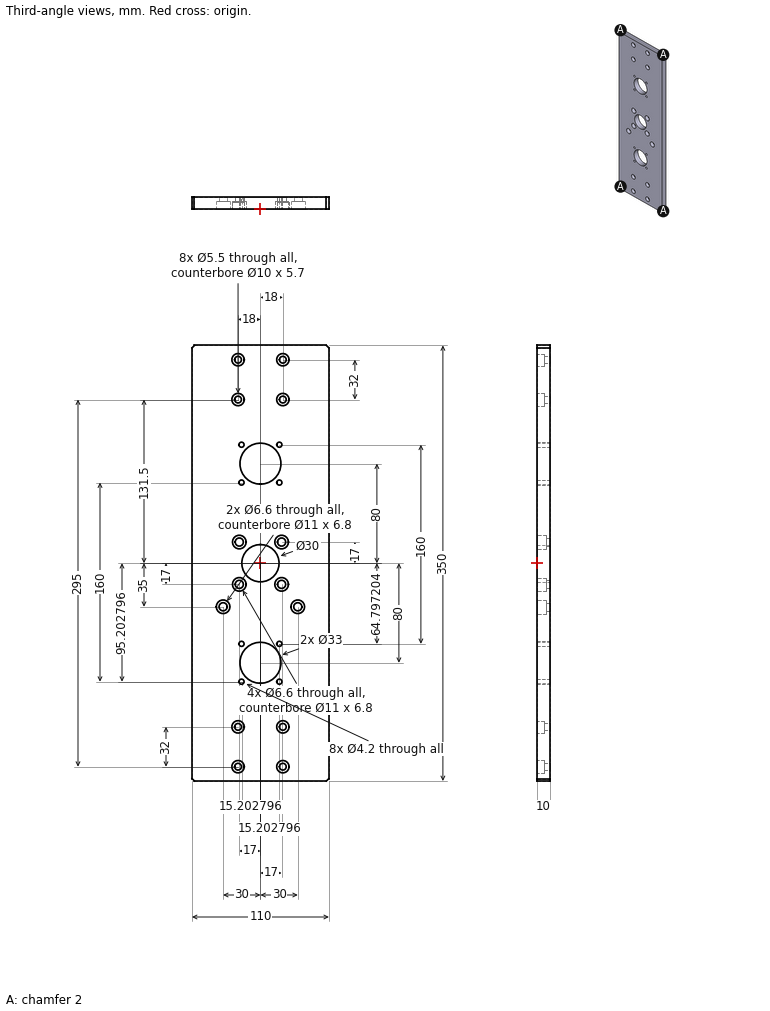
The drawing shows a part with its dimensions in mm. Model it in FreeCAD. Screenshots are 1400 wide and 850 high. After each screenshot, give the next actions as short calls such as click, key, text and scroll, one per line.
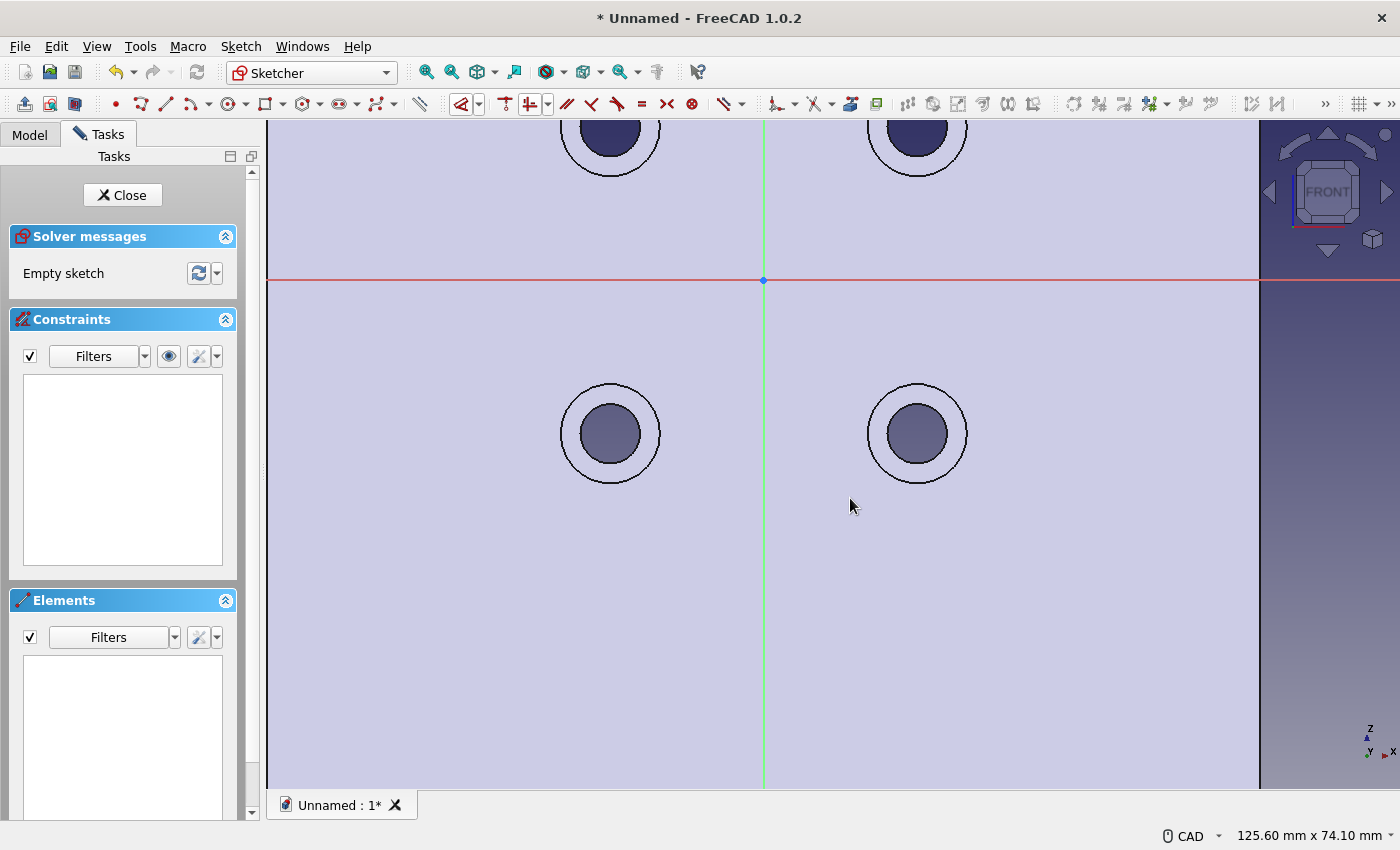
key(g)
key(c)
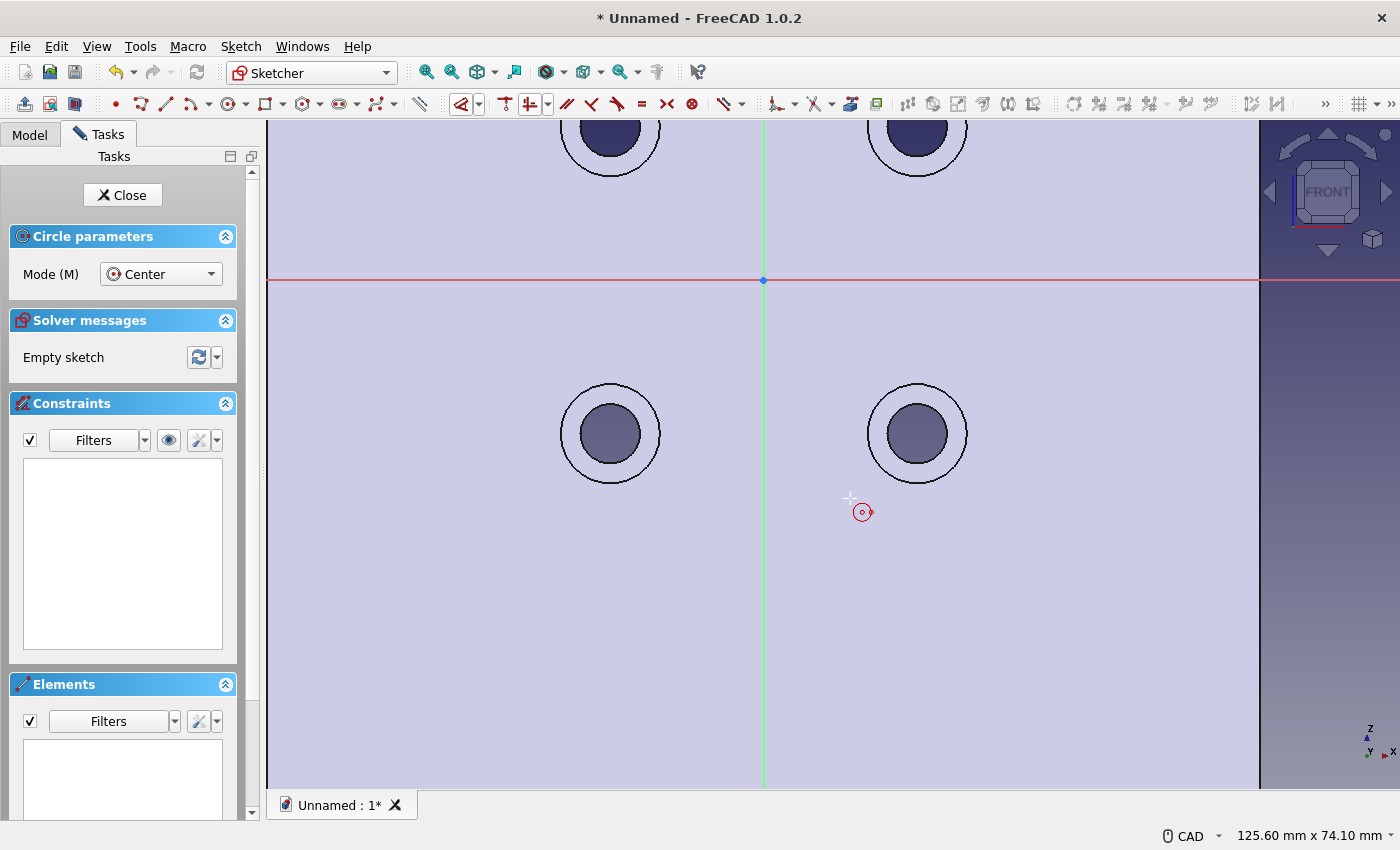
click(493, 596)
move(514, 575)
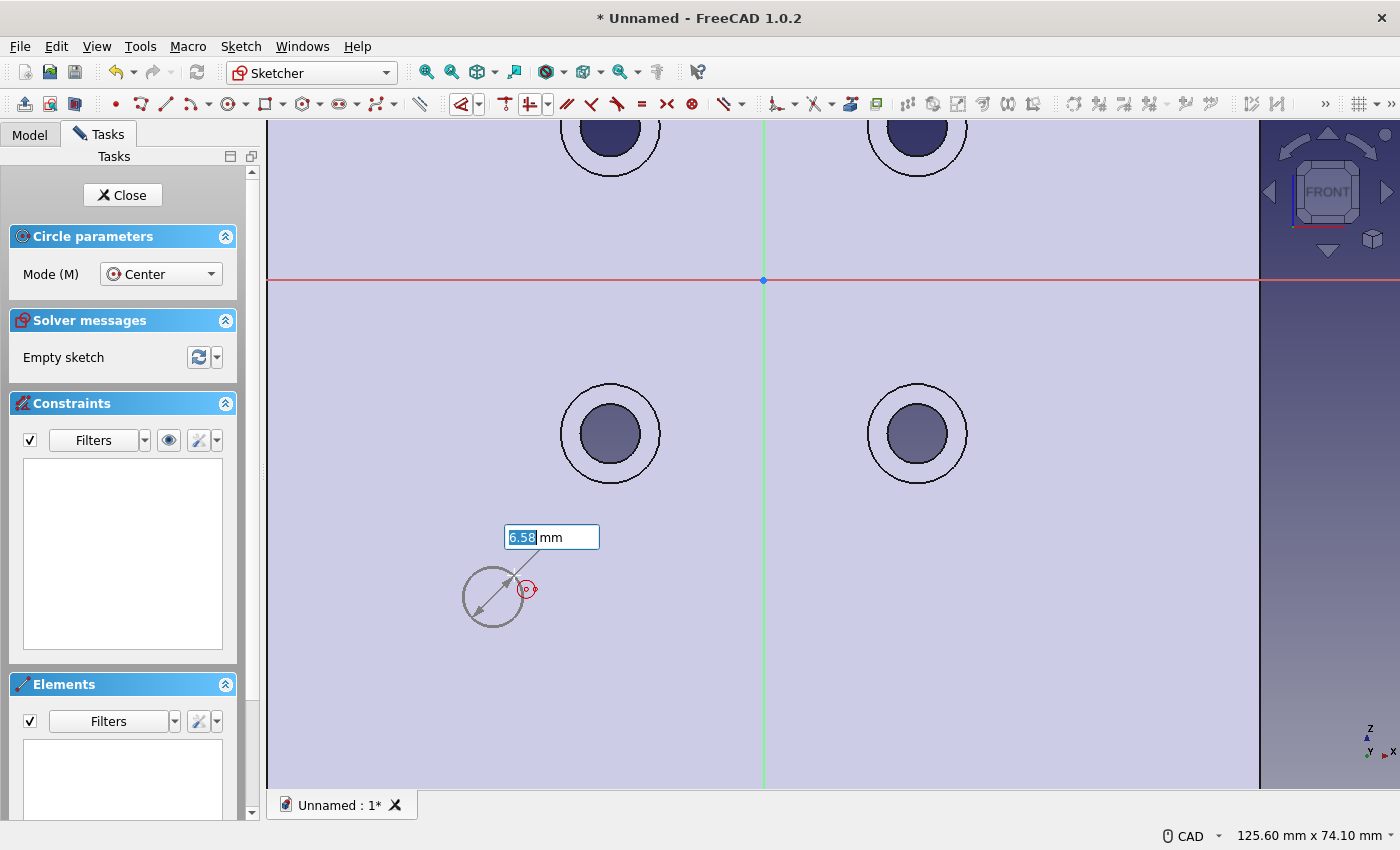
text(6.6)
key(Return)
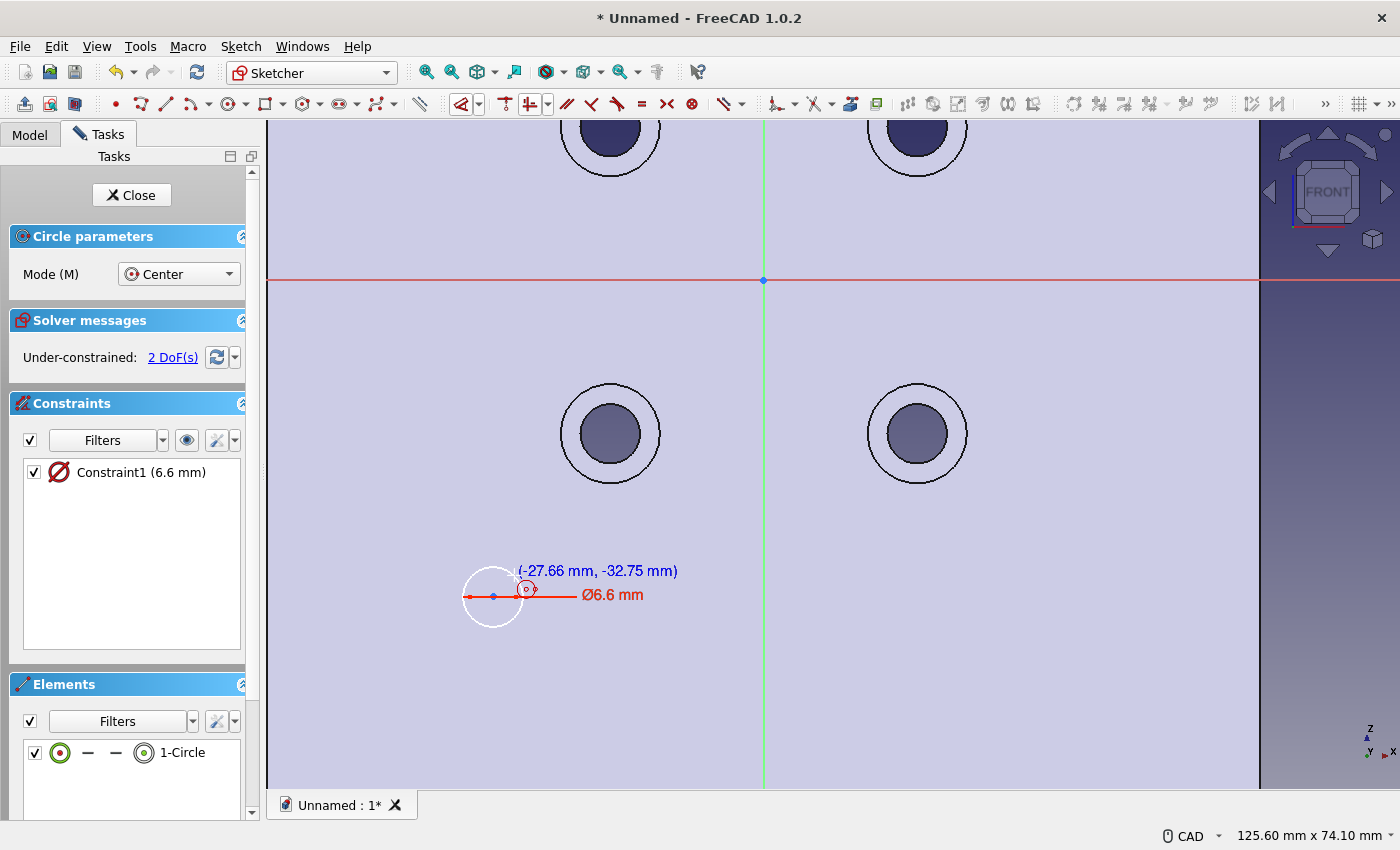
click(1035, 596)
move(1056, 575)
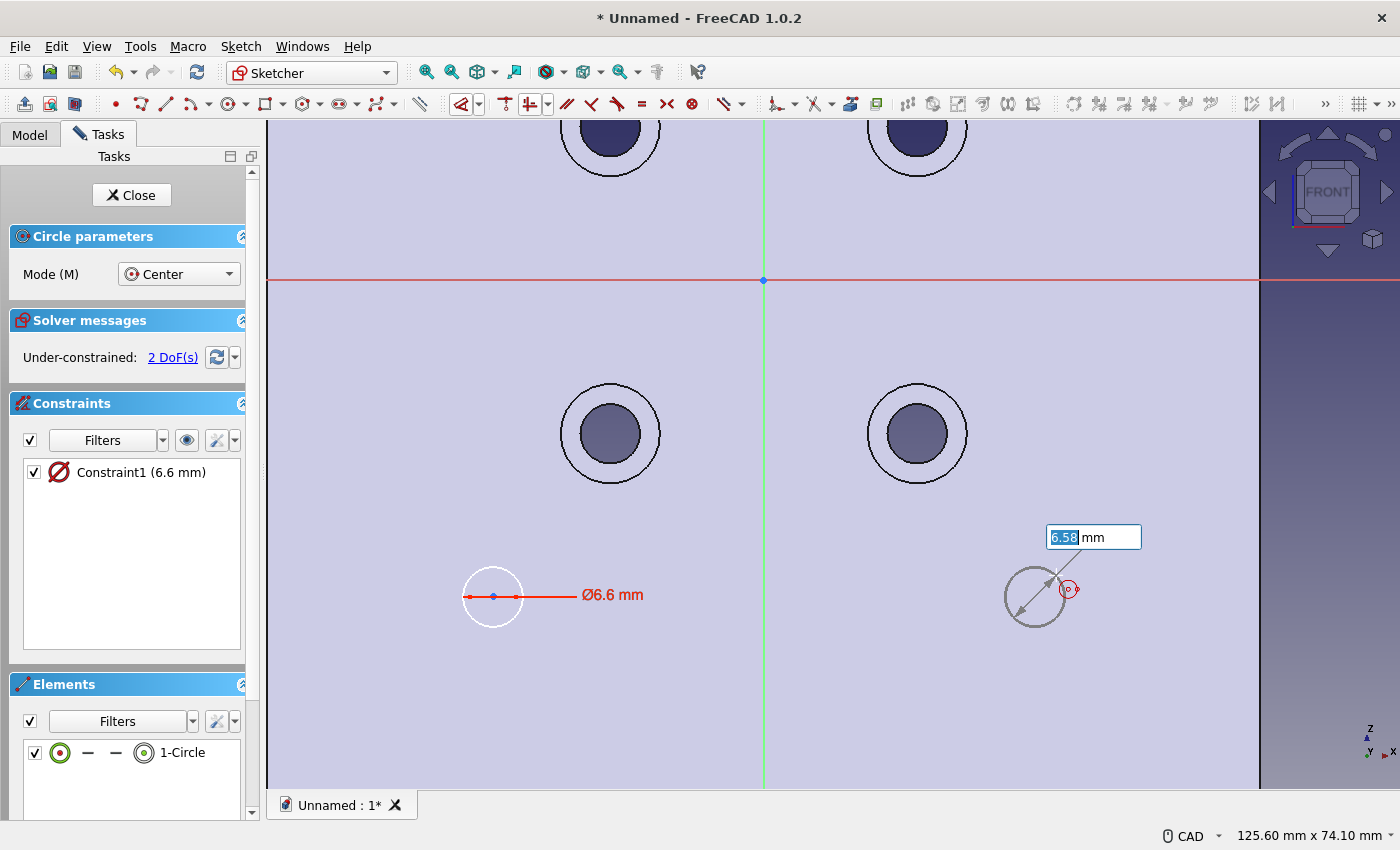
text(6.6)
key(Return)
key(Escape)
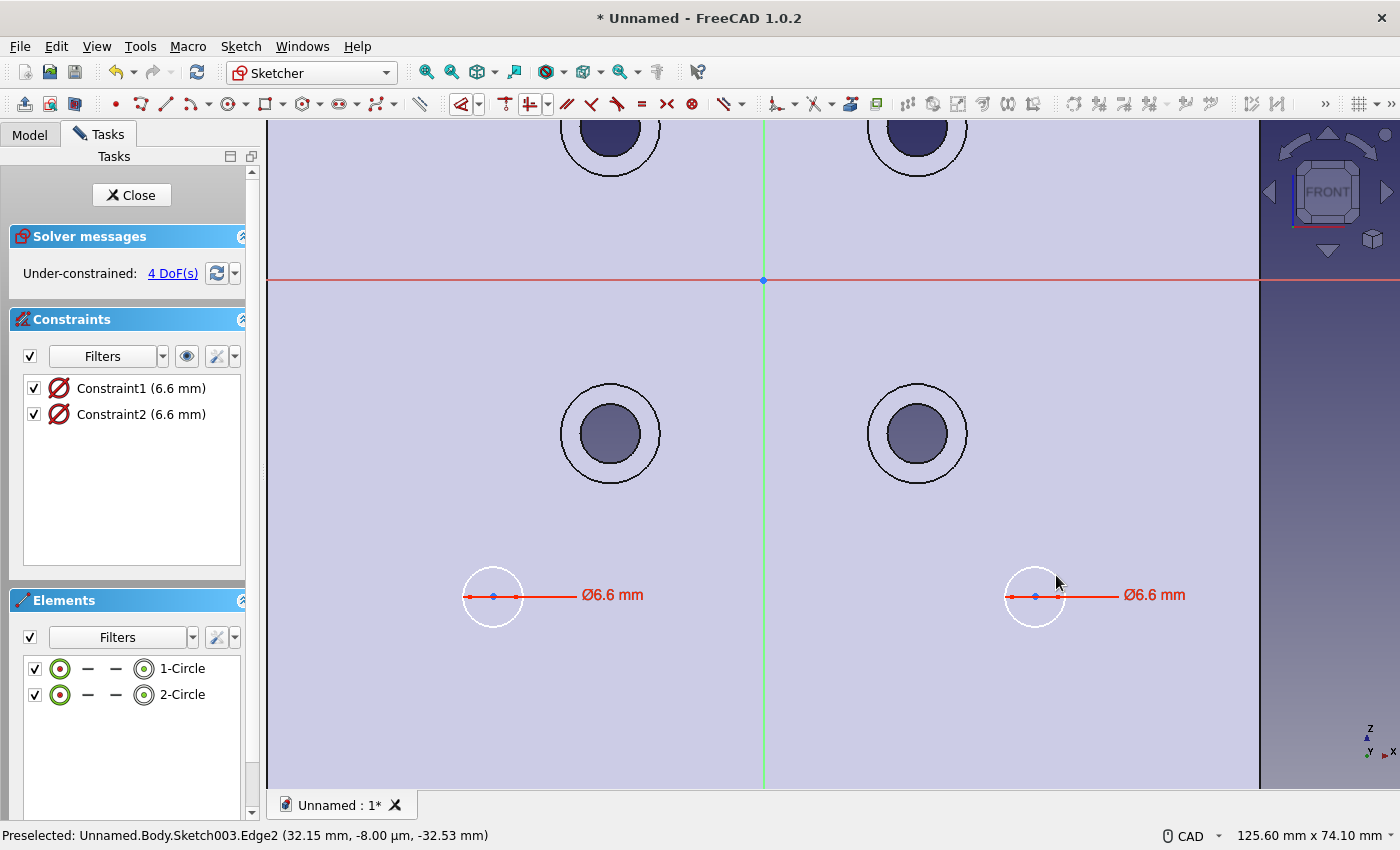
click(493, 597)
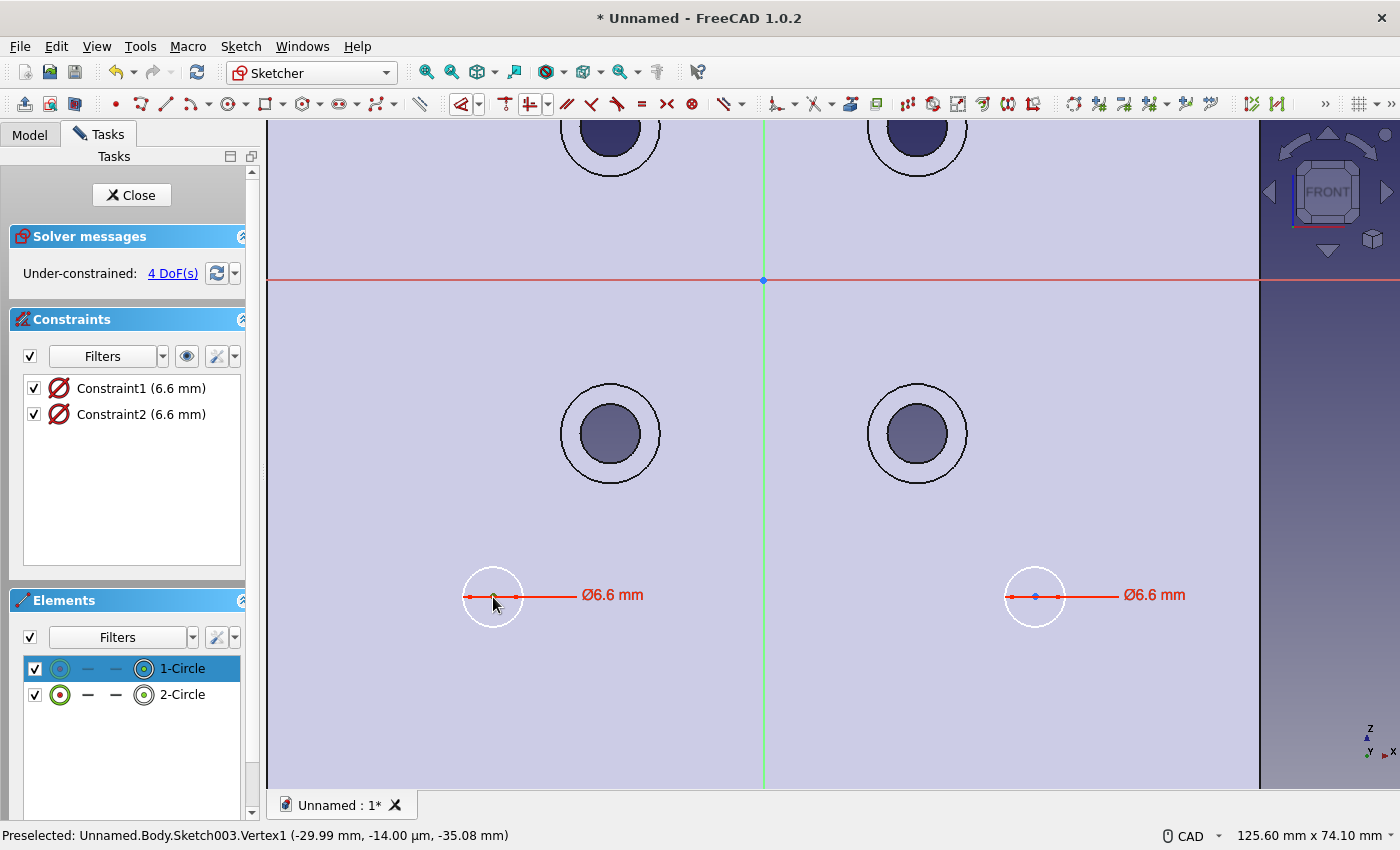
click(1035, 597)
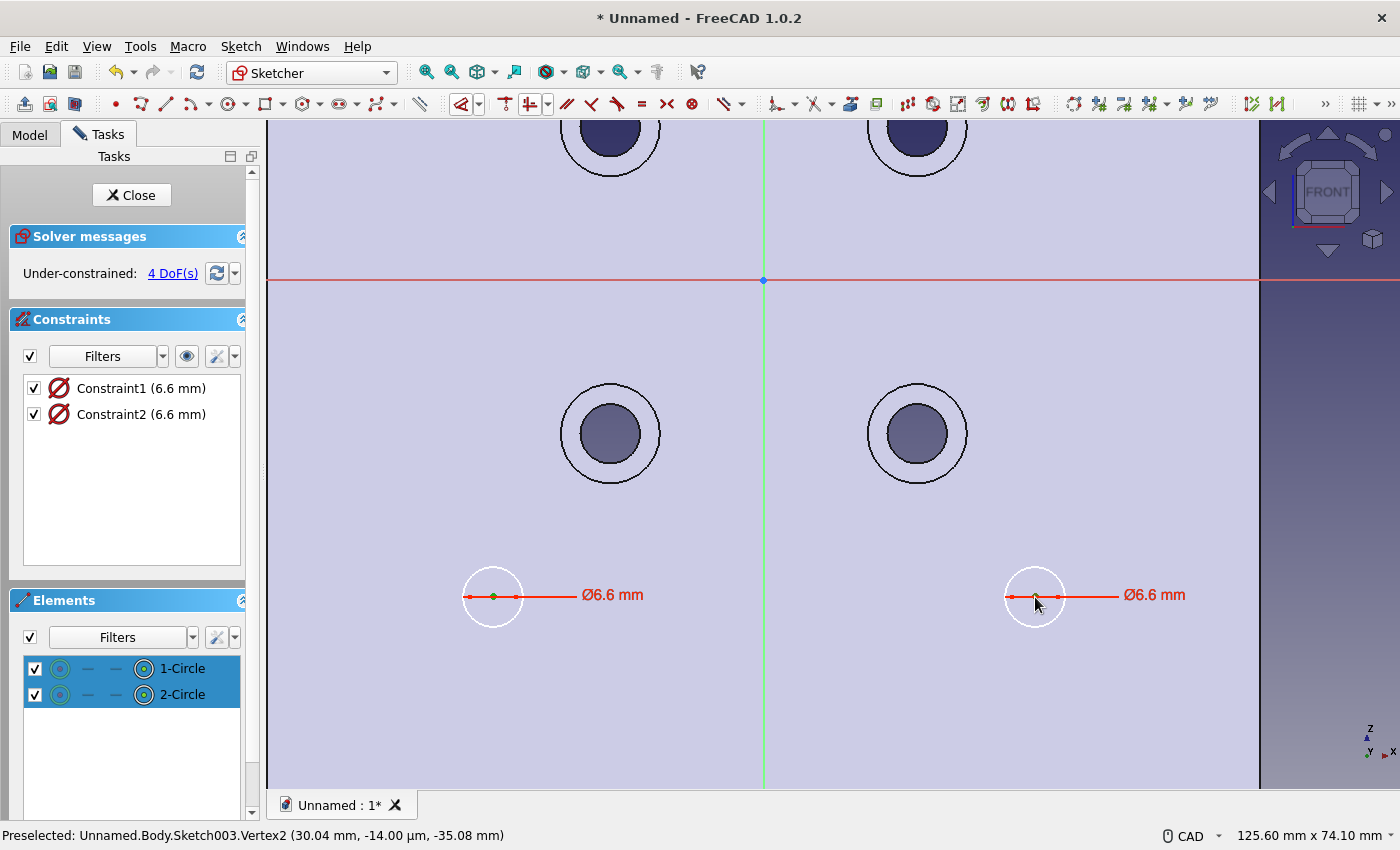
key(h)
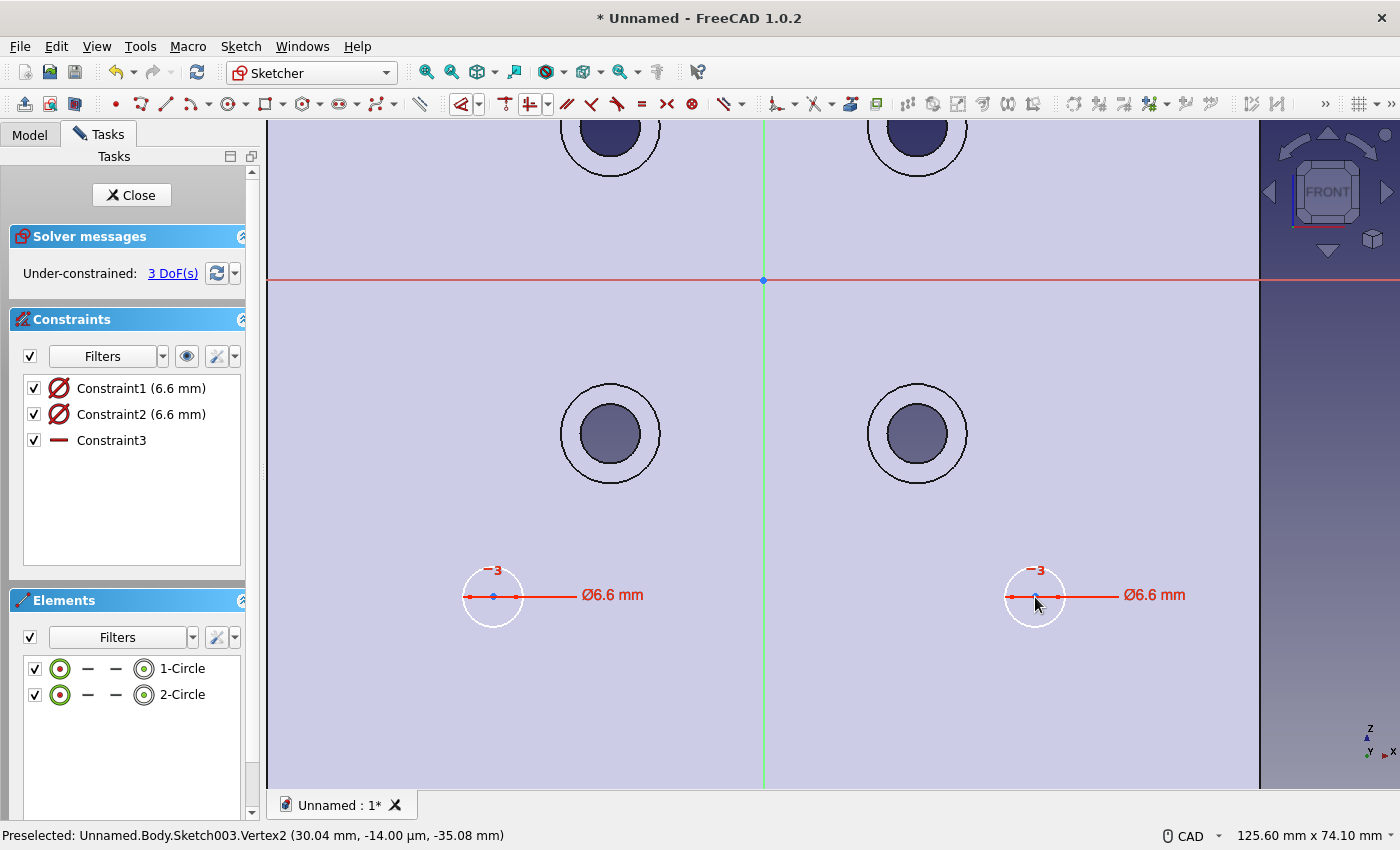
click(493, 597)